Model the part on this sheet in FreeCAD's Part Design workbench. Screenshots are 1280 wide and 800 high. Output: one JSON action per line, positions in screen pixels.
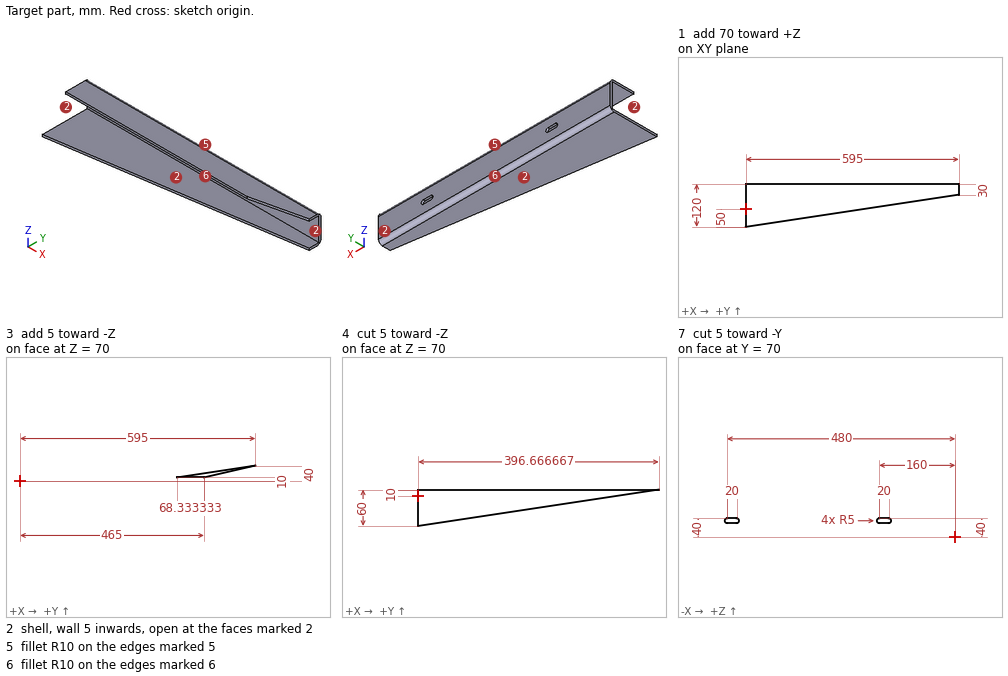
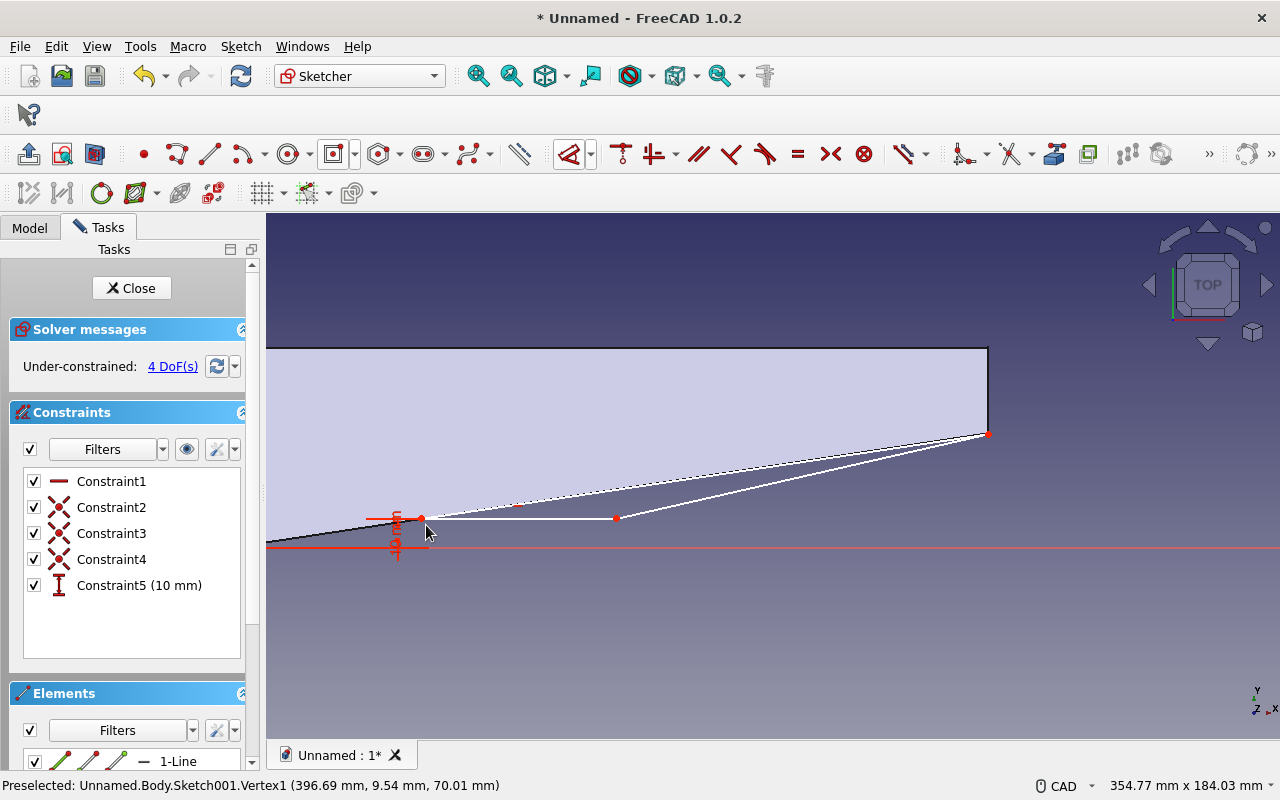
{"action": "left_click", "coordinate": [988, 434]}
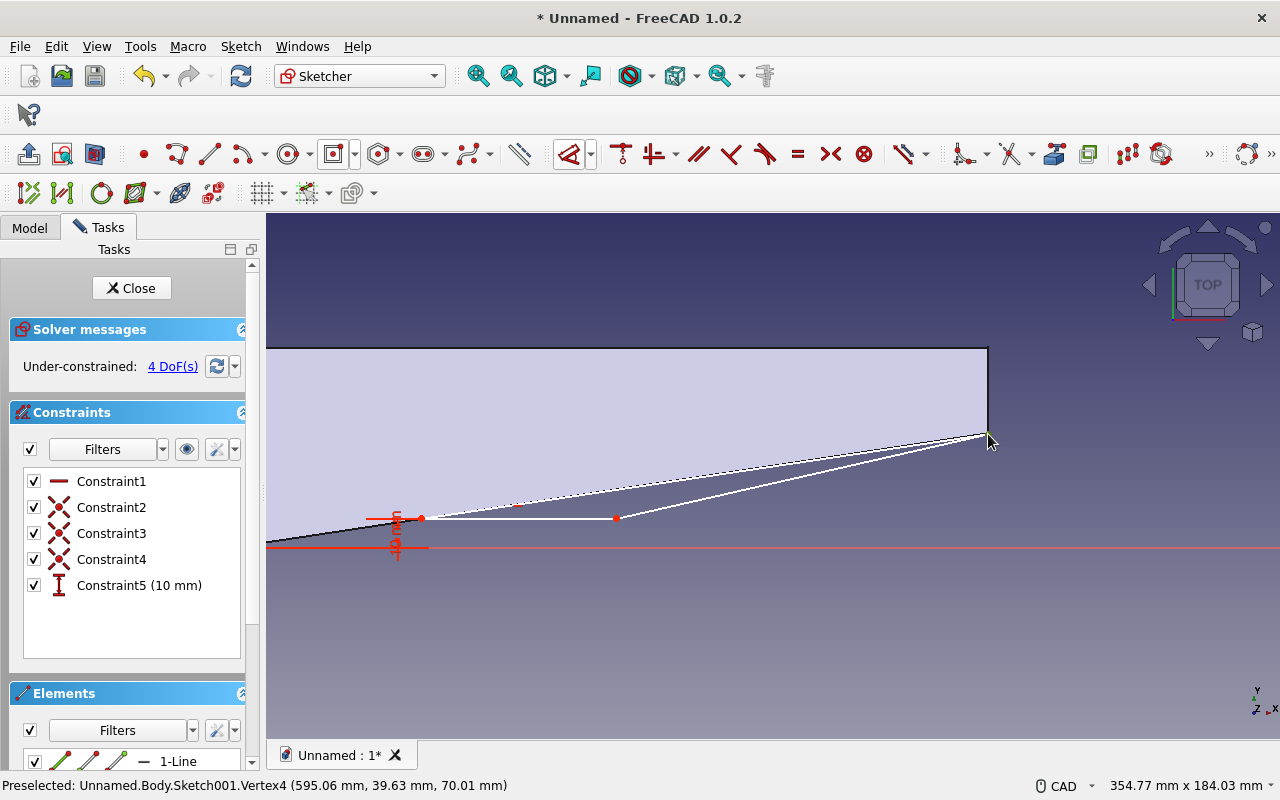
{"action": "key", "text": "i"}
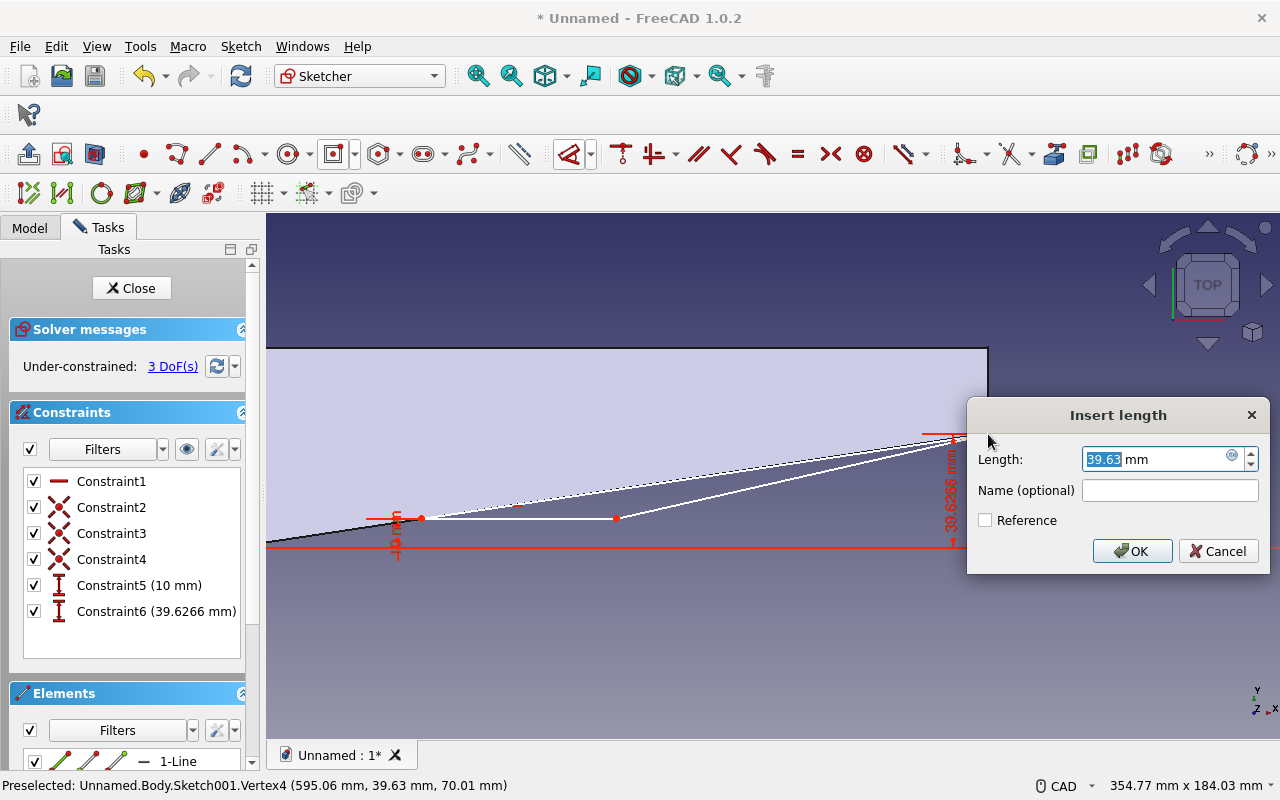
{"action": "type", "text": "40"}
{"action": "key", "text": "Return"}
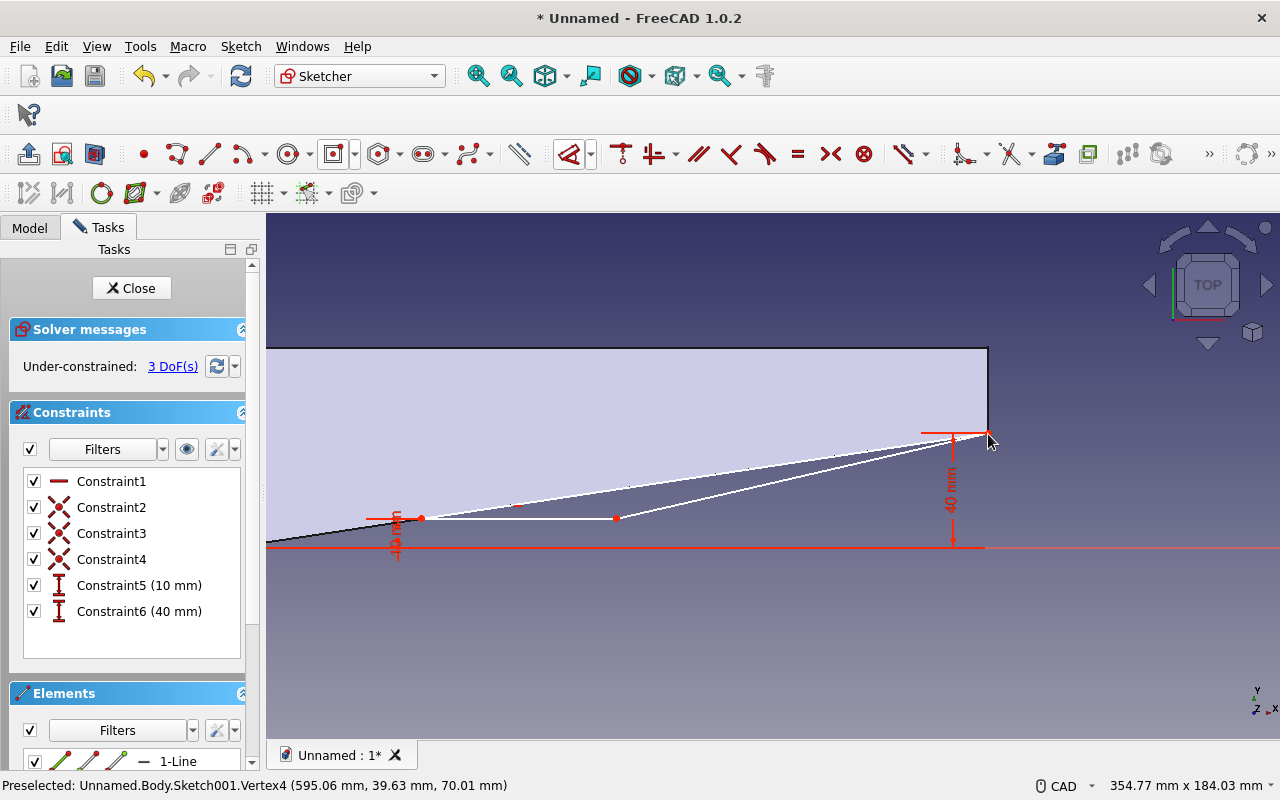
{"action": "left_click", "coordinate": [616, 519]}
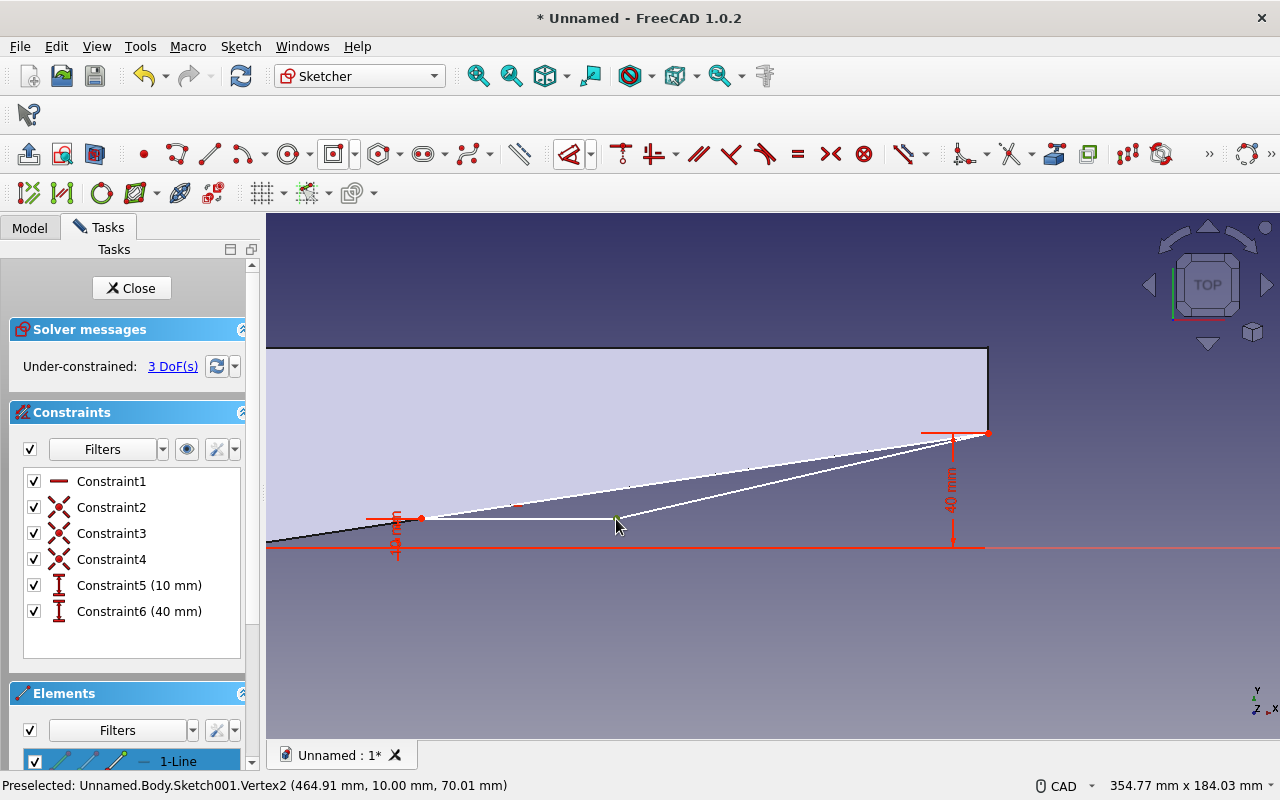
{"action": "left_click", "coordinate": [590, 154]}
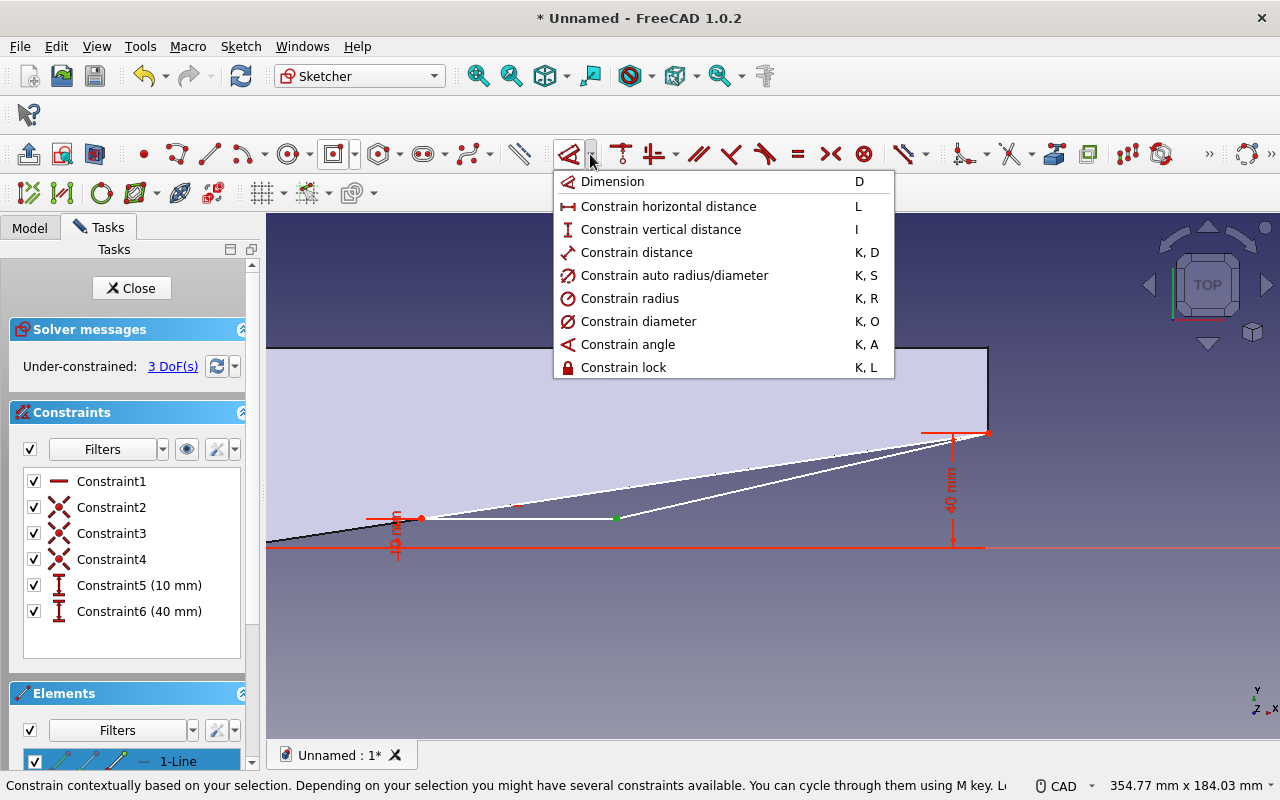
{"action": "left_click", "coordinate": [724, 206]}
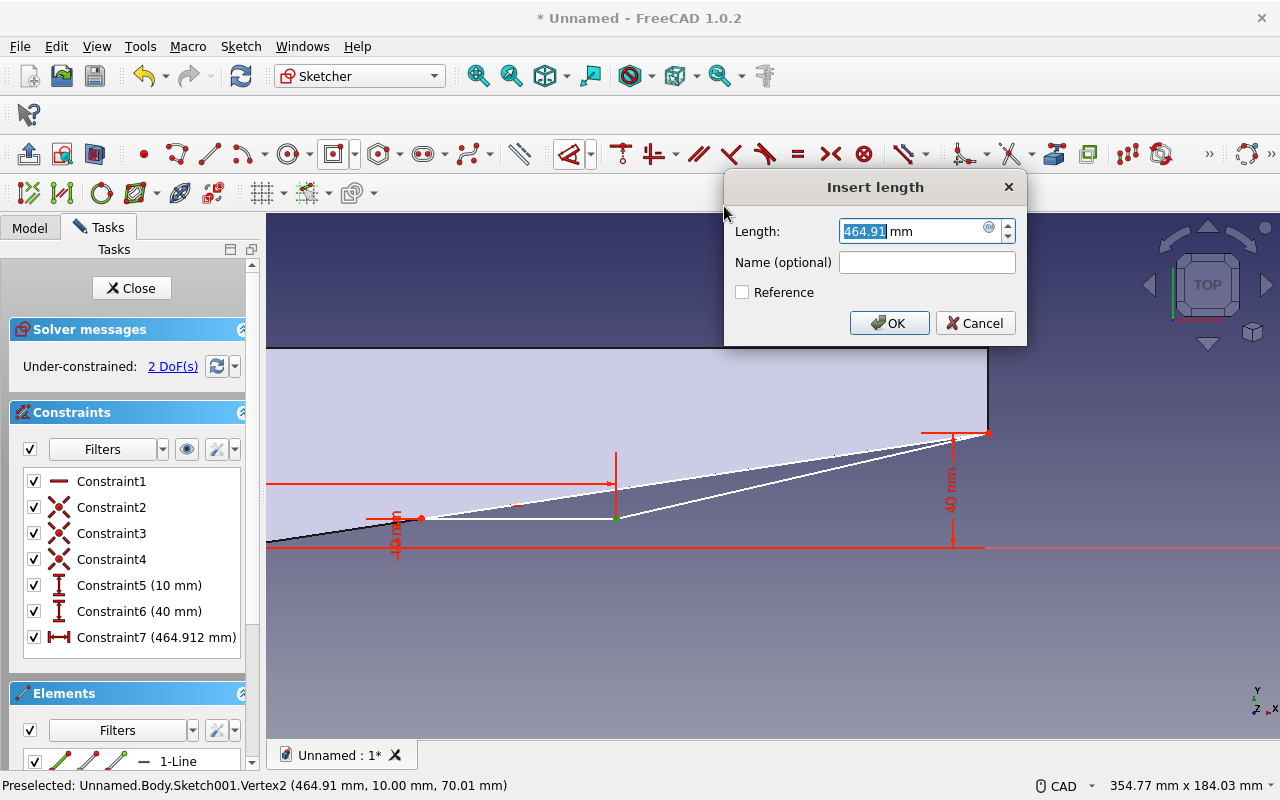
{"action": "type", "text": "465"}
{"action": "key", "text": "Return"}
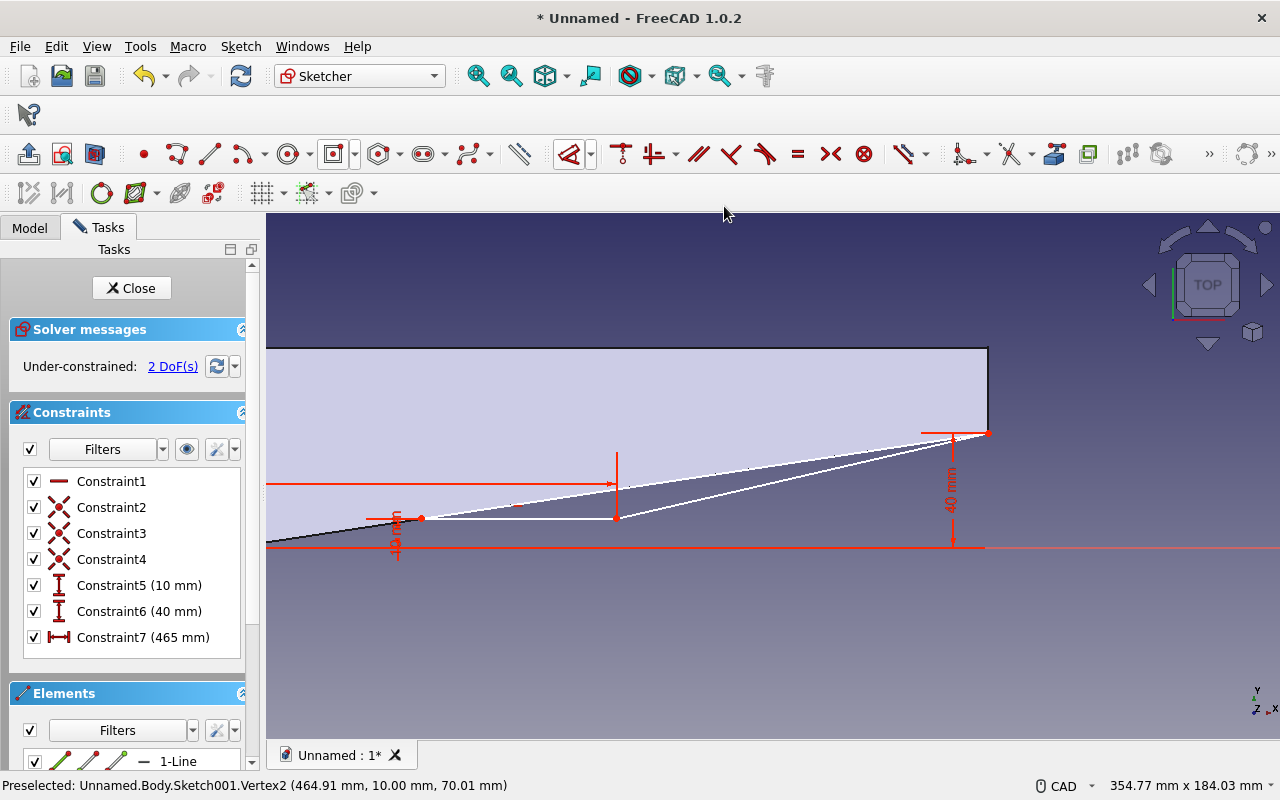
{"action": "left_click", "coordinate": [988, 433]}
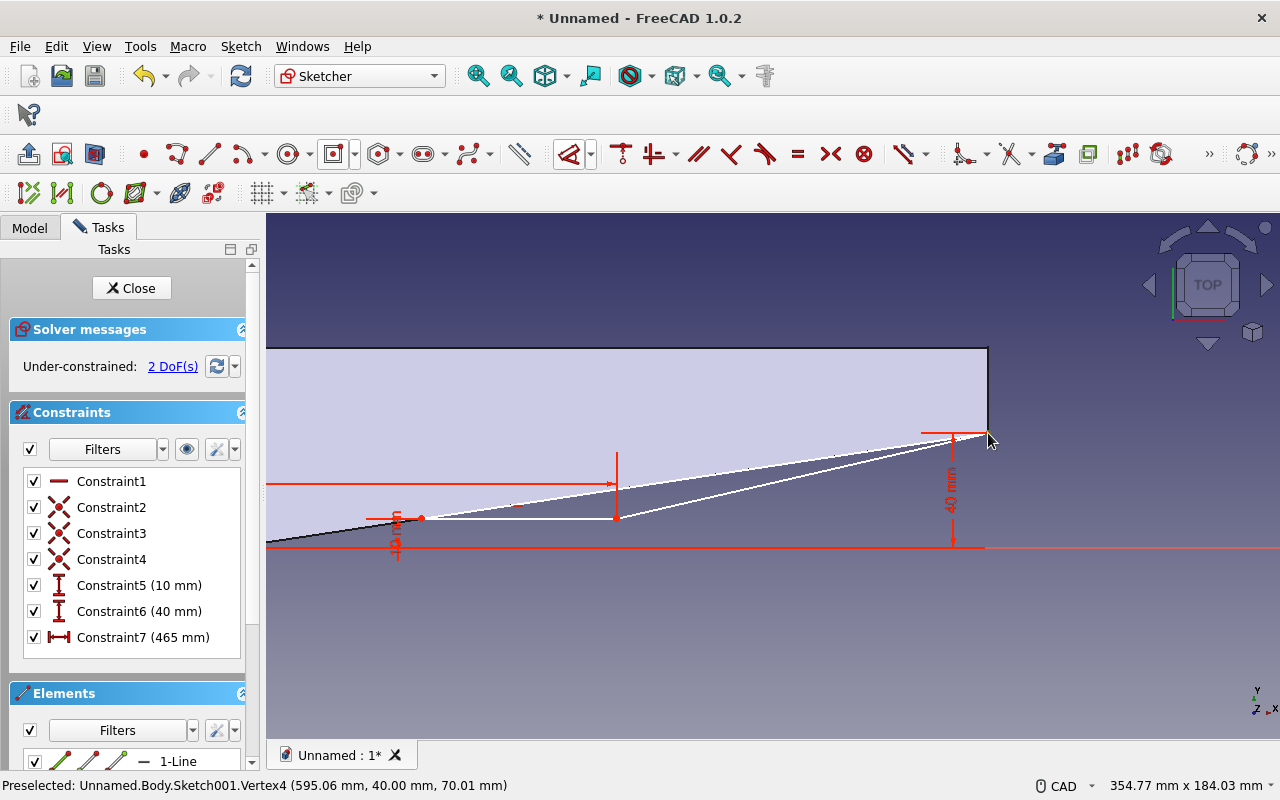
{"action": "left_click", "coordinate": [590, 154]}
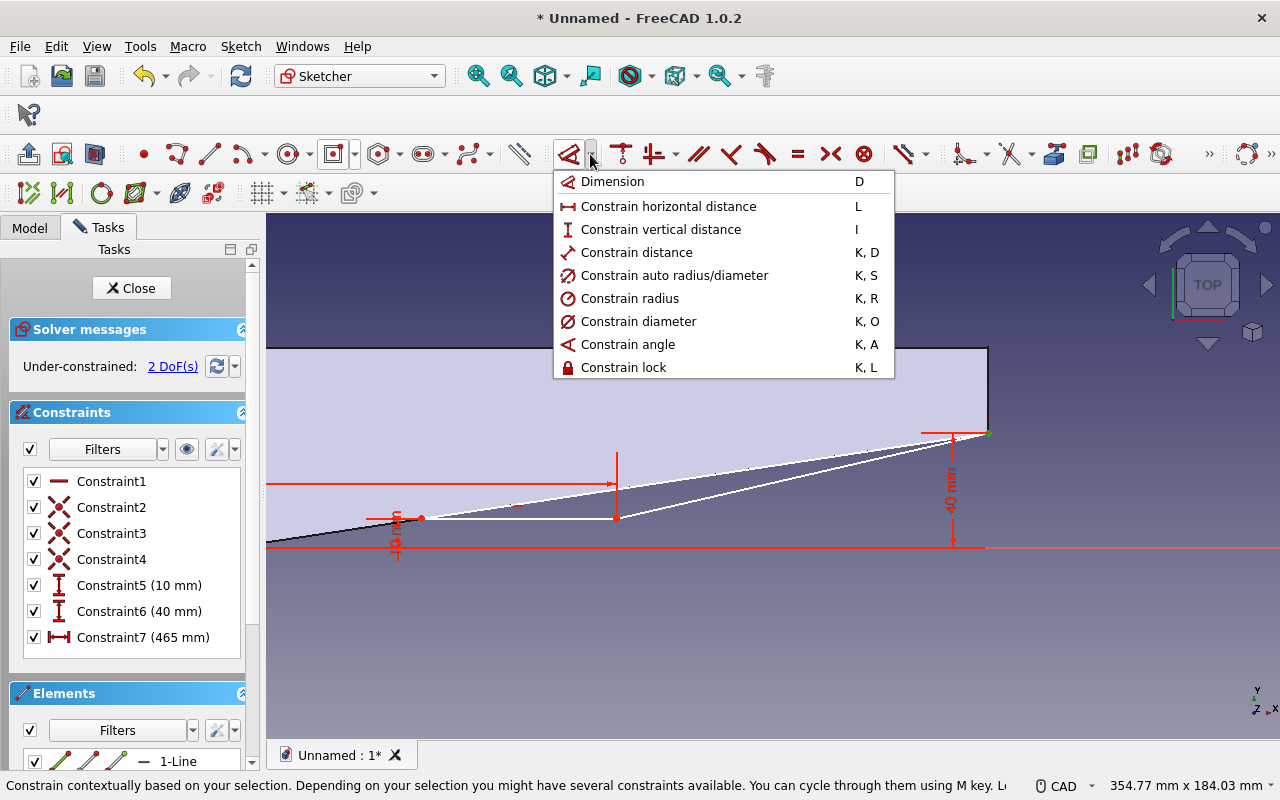
{"action": "left_click", "coordinate": [724, 206]}